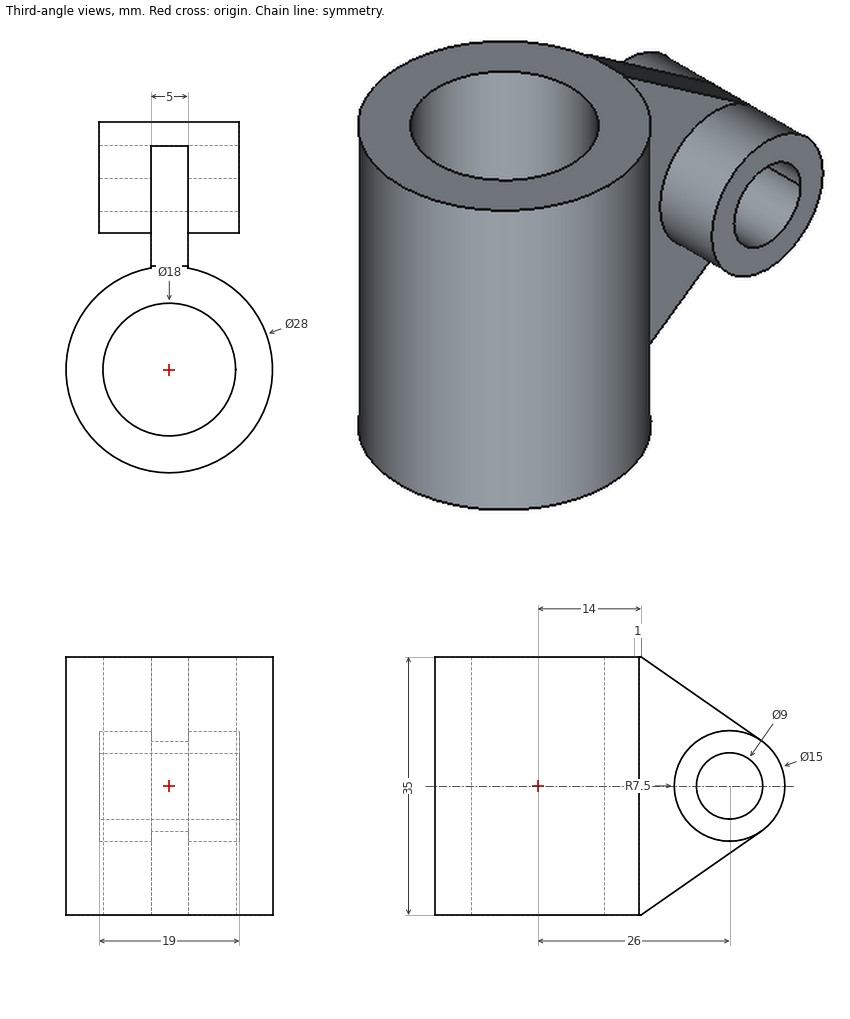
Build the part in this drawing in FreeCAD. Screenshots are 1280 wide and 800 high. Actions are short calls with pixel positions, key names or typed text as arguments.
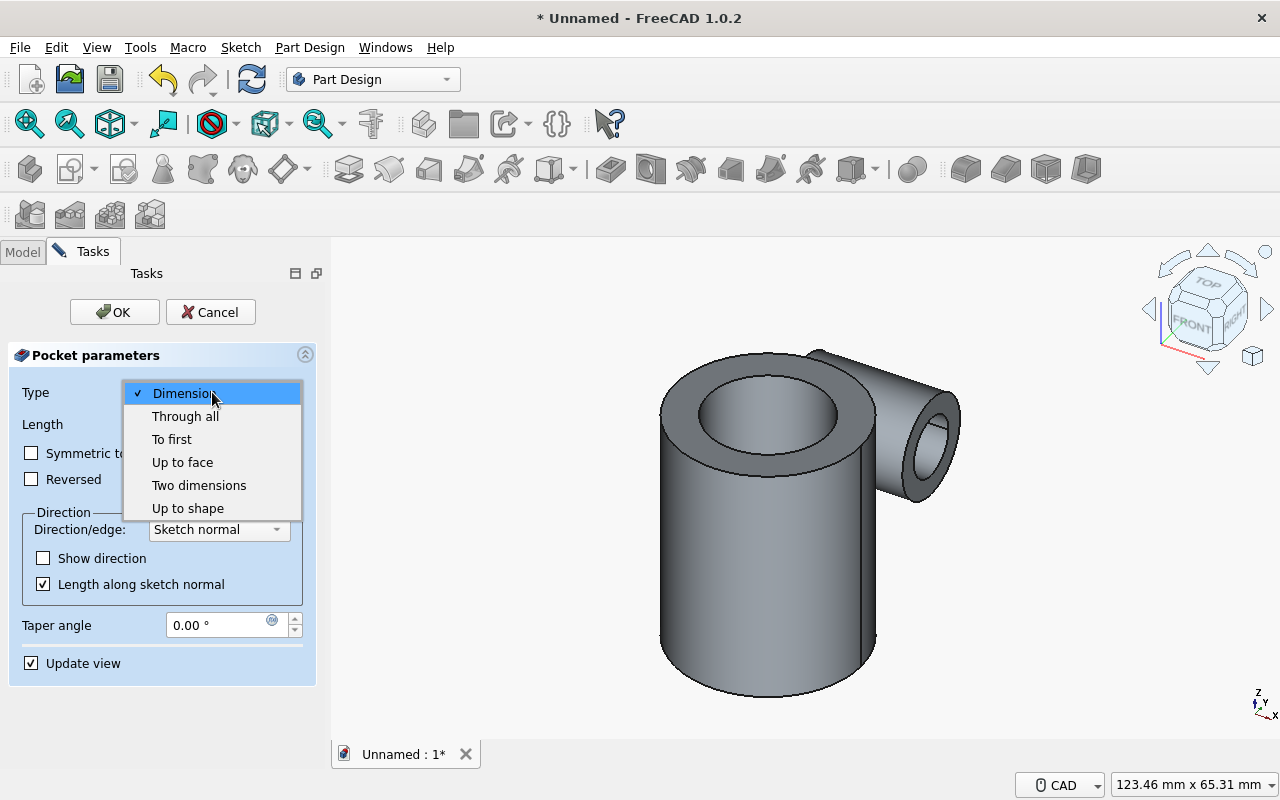
click(212, 416)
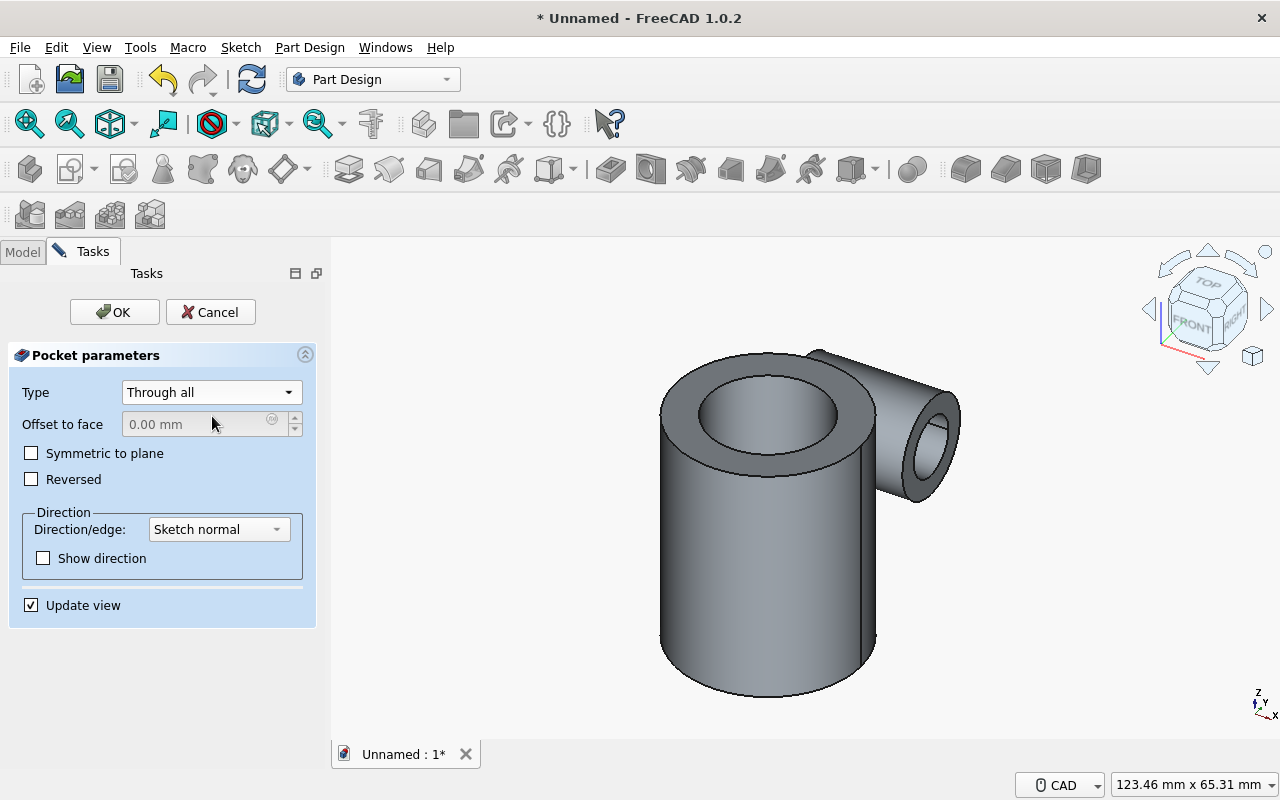
click(115, 312)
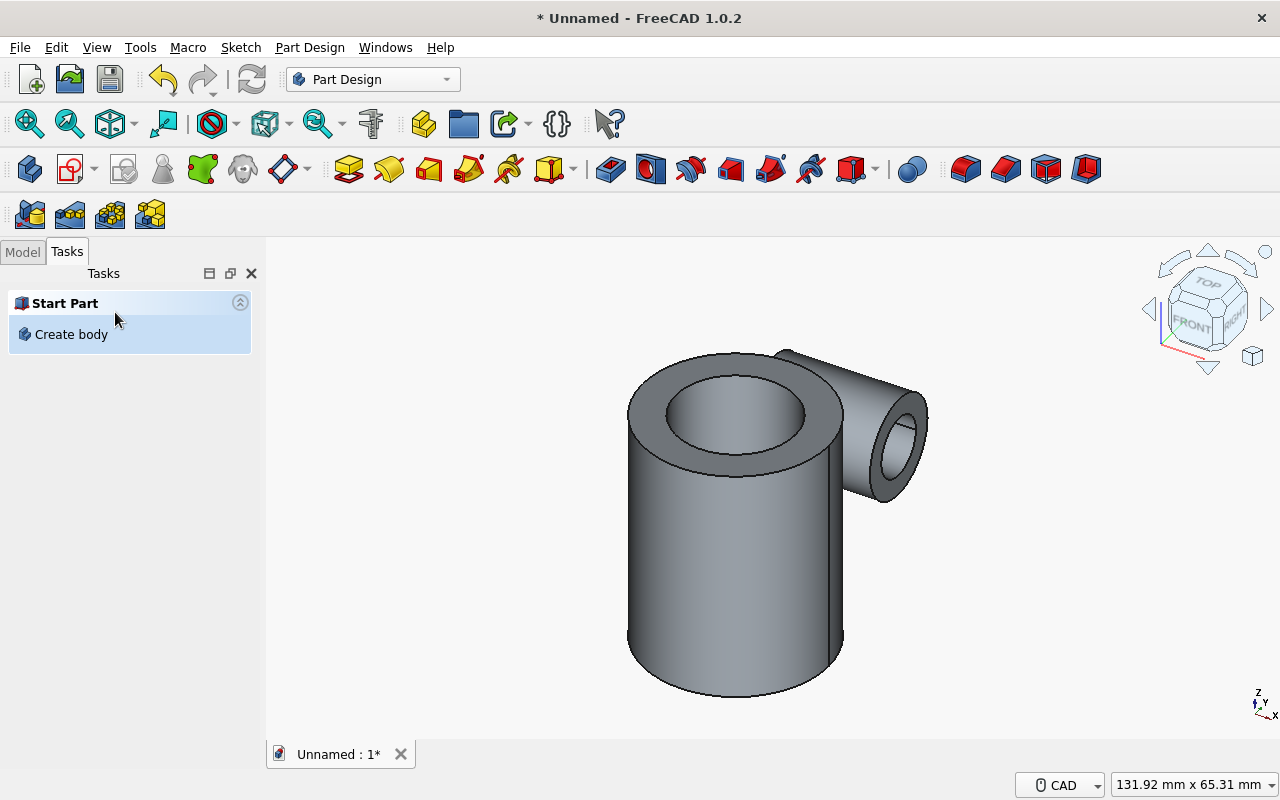
key(v)
key(f)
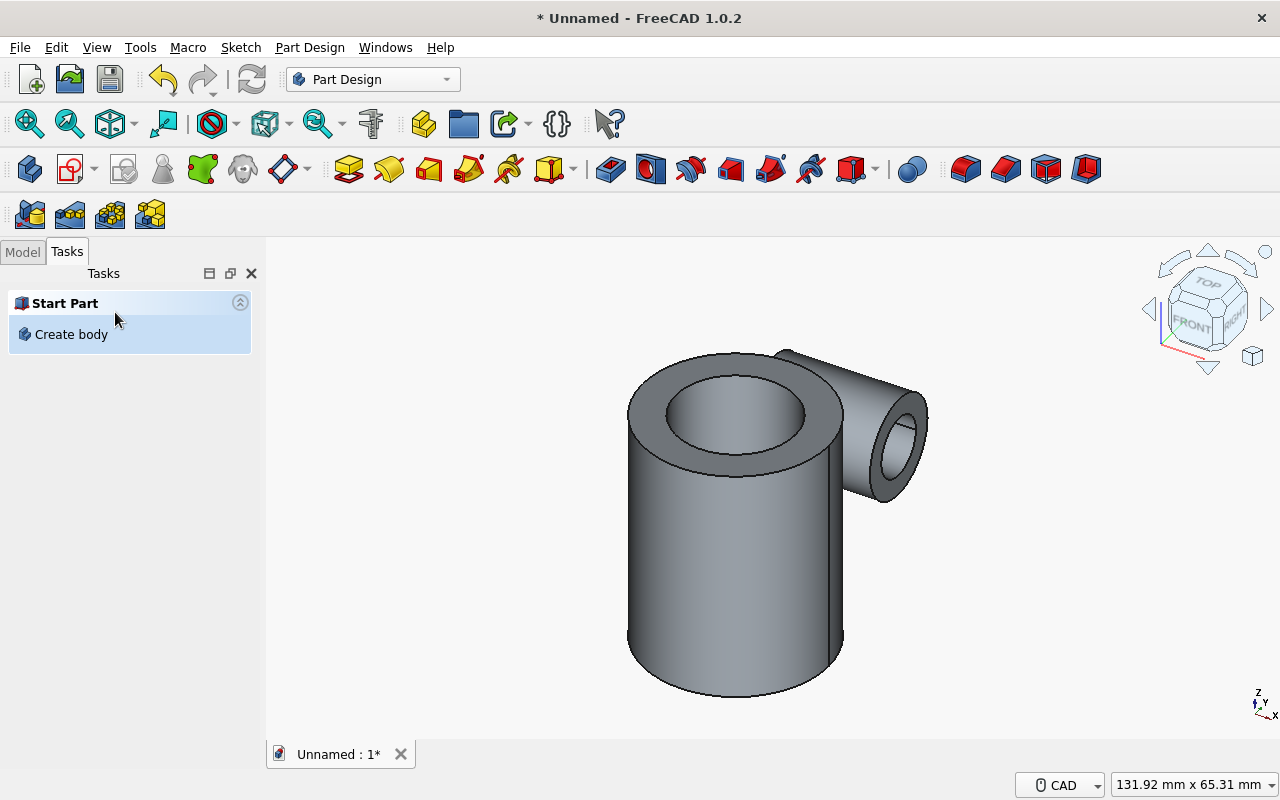
click(23, 251)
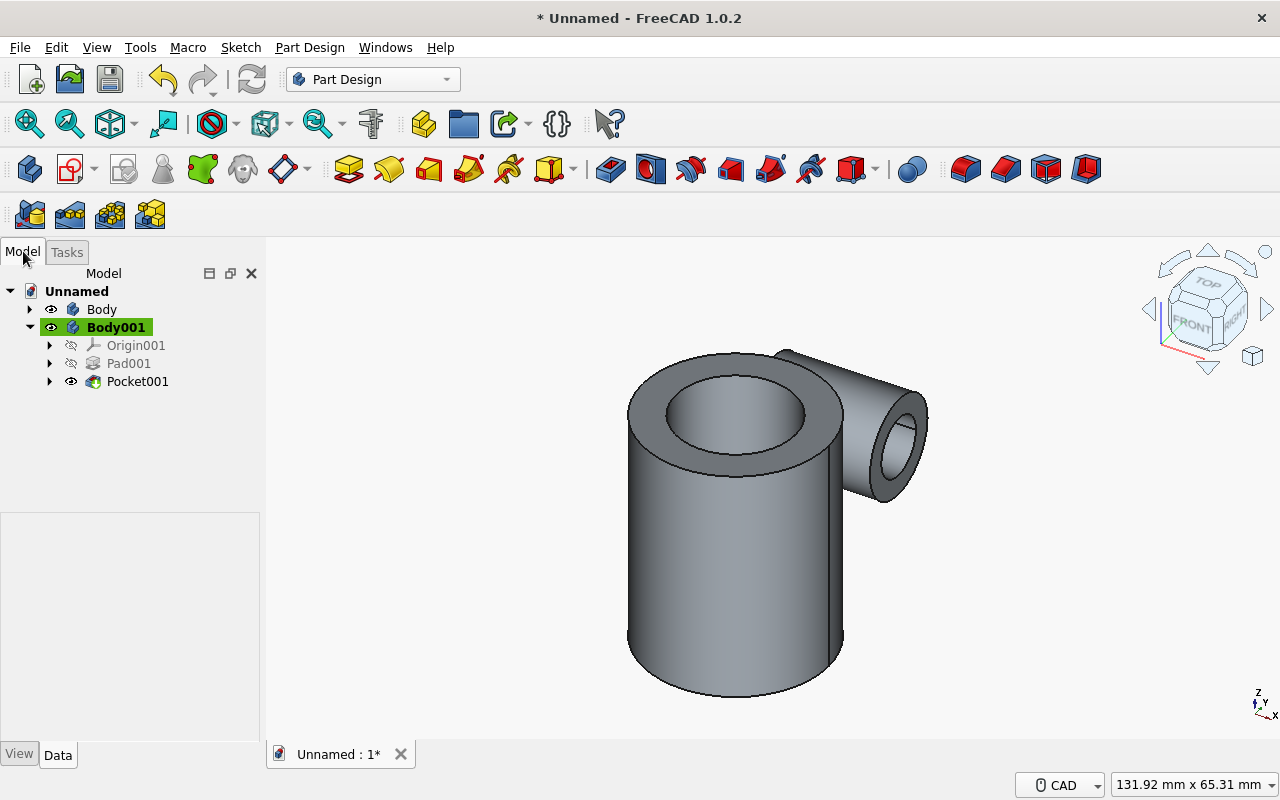
double_click(96, 309)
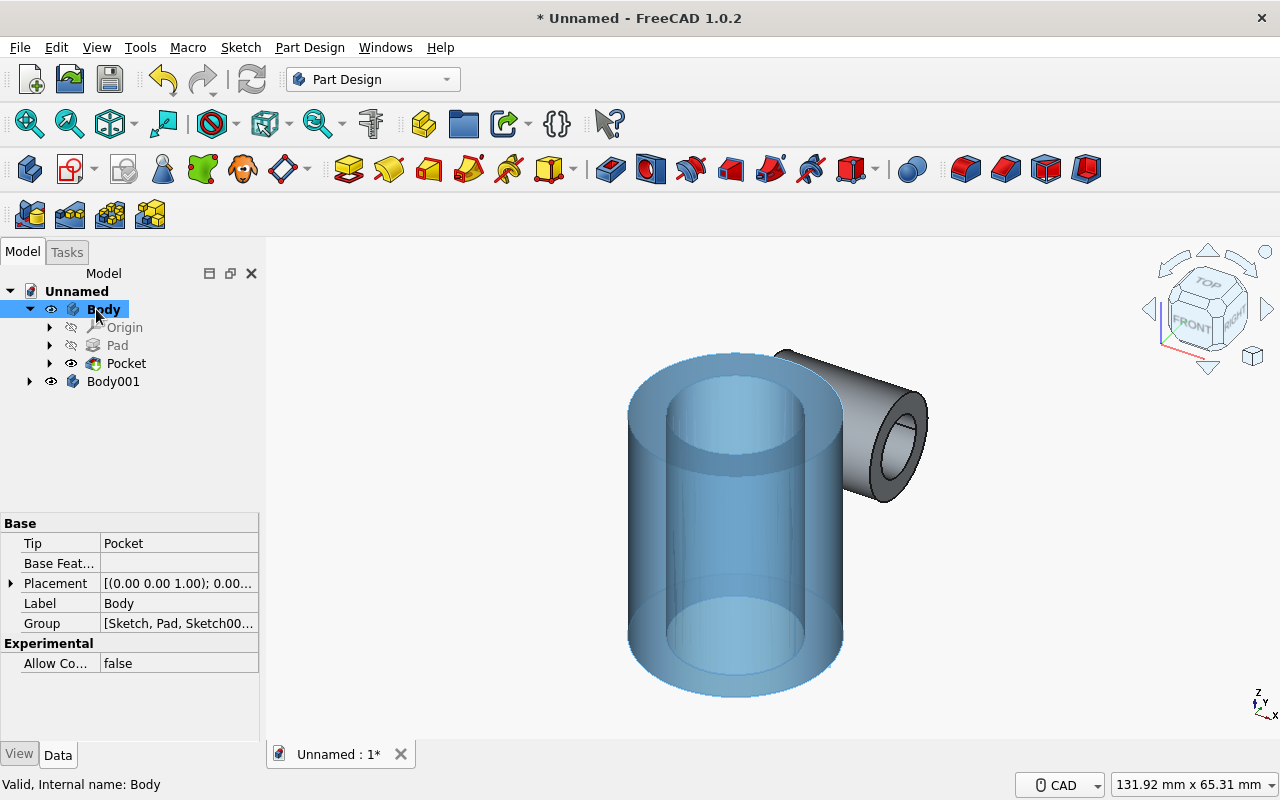
click(96, 309)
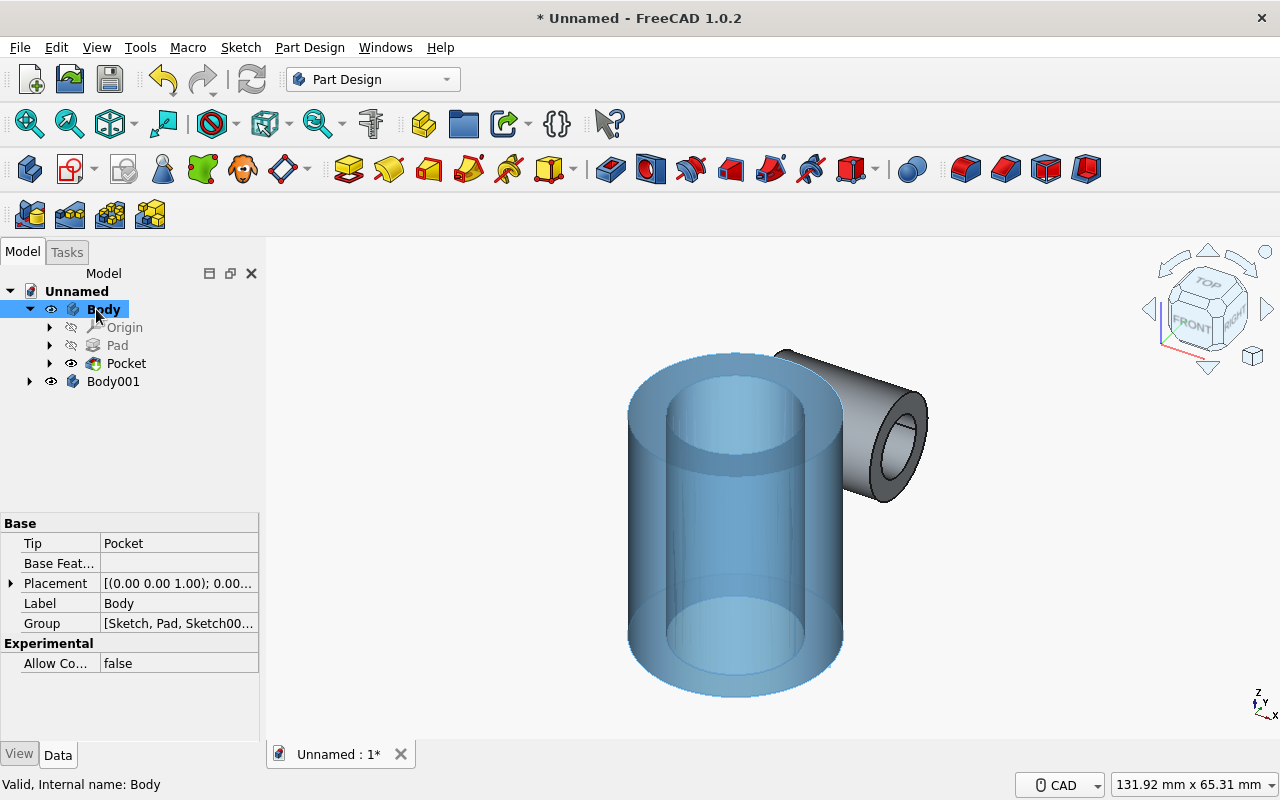
click(146, 663)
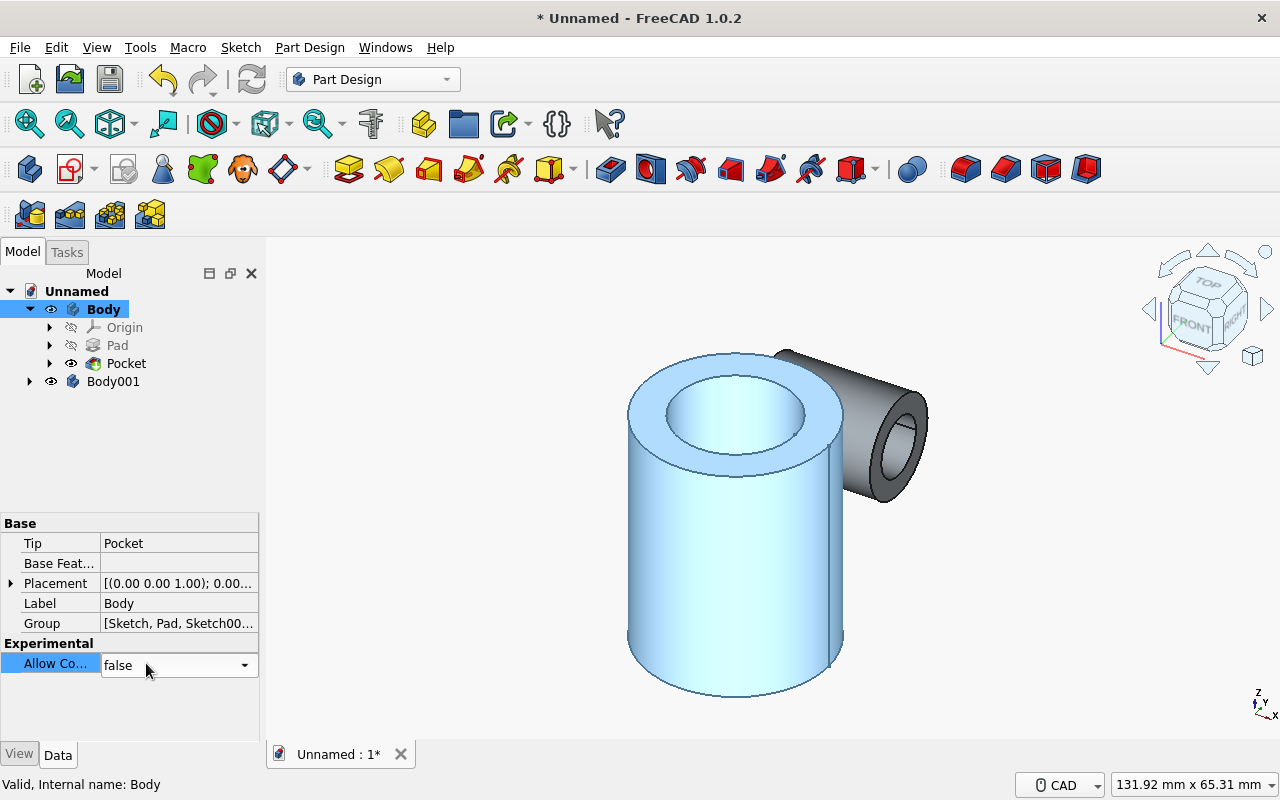
click(146, 663)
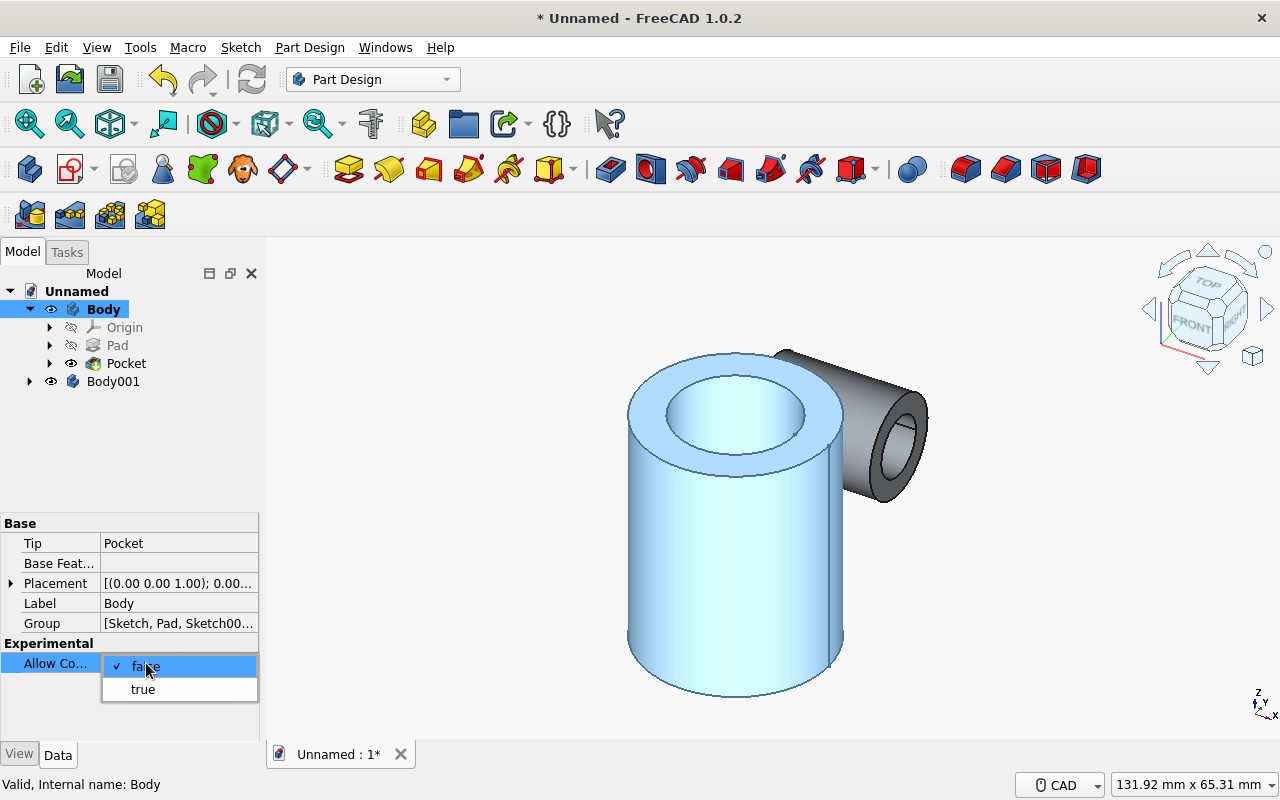
click(179, 690)
key(Return)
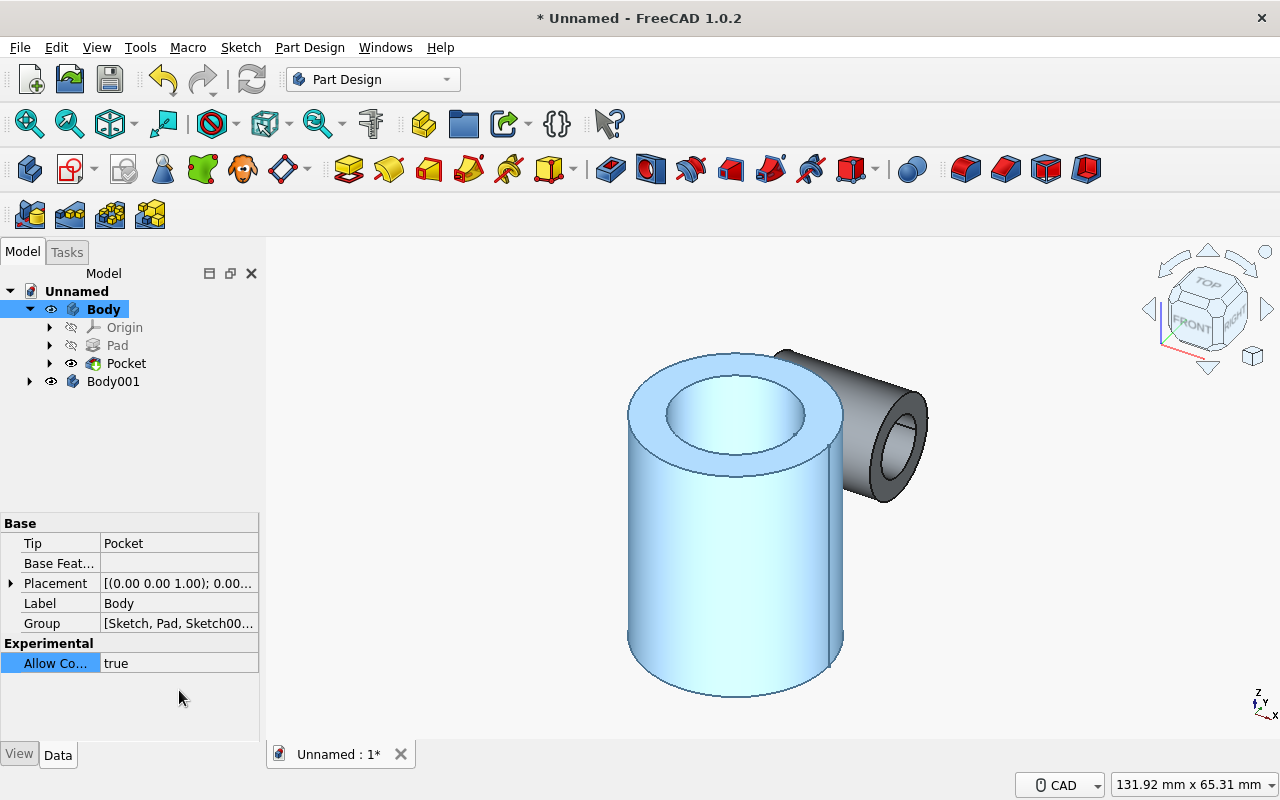
click(96, 381)